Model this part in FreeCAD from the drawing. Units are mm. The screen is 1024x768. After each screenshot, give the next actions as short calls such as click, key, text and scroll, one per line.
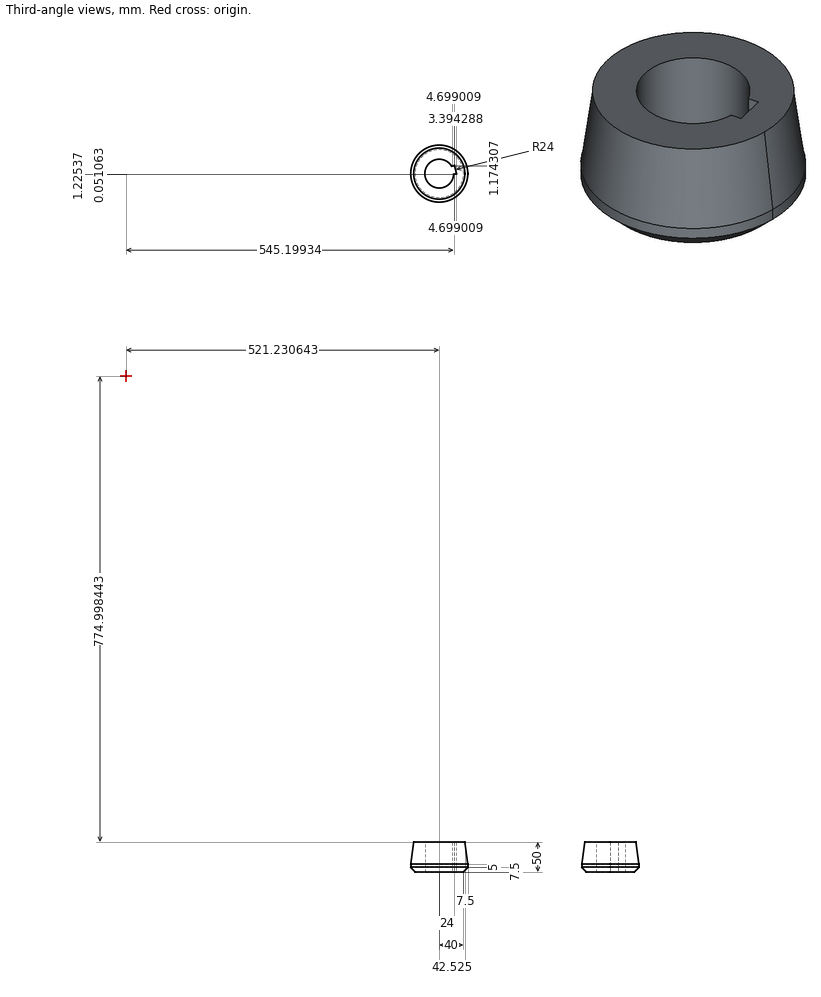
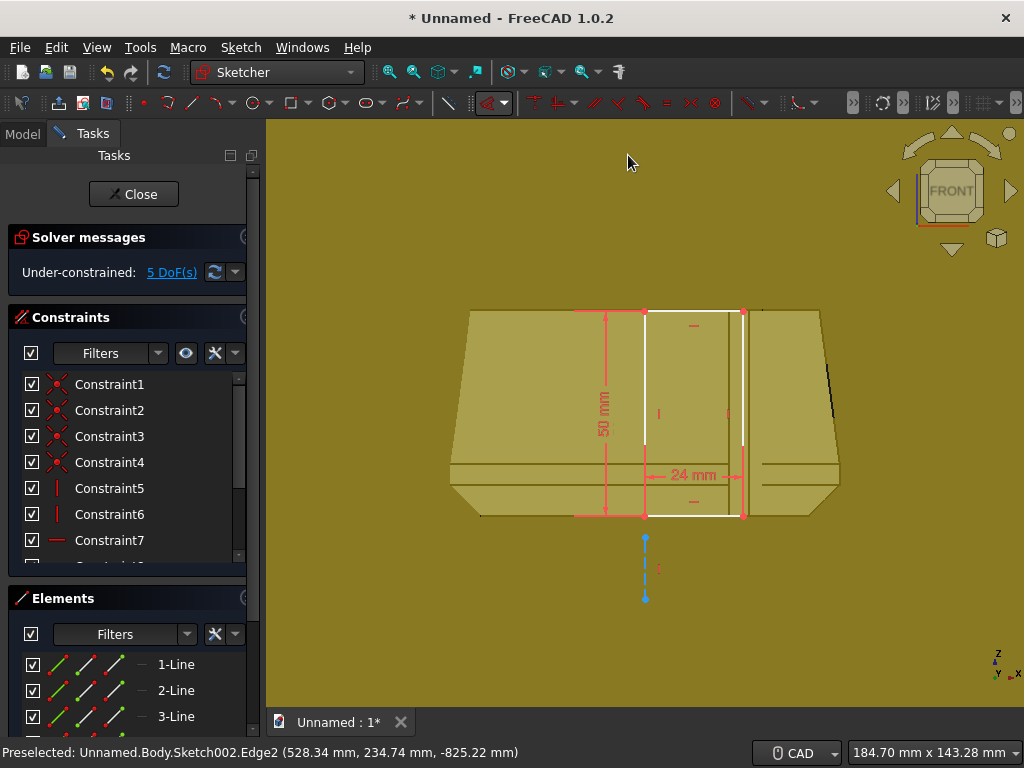
click(645, 311)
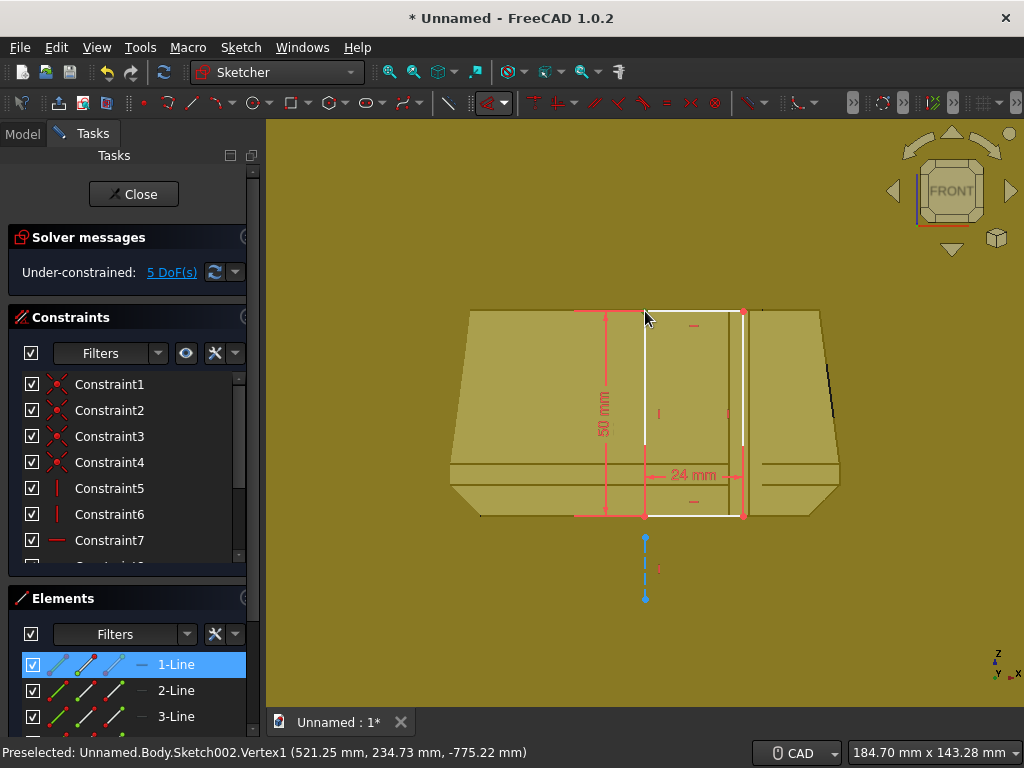
click(506, 104)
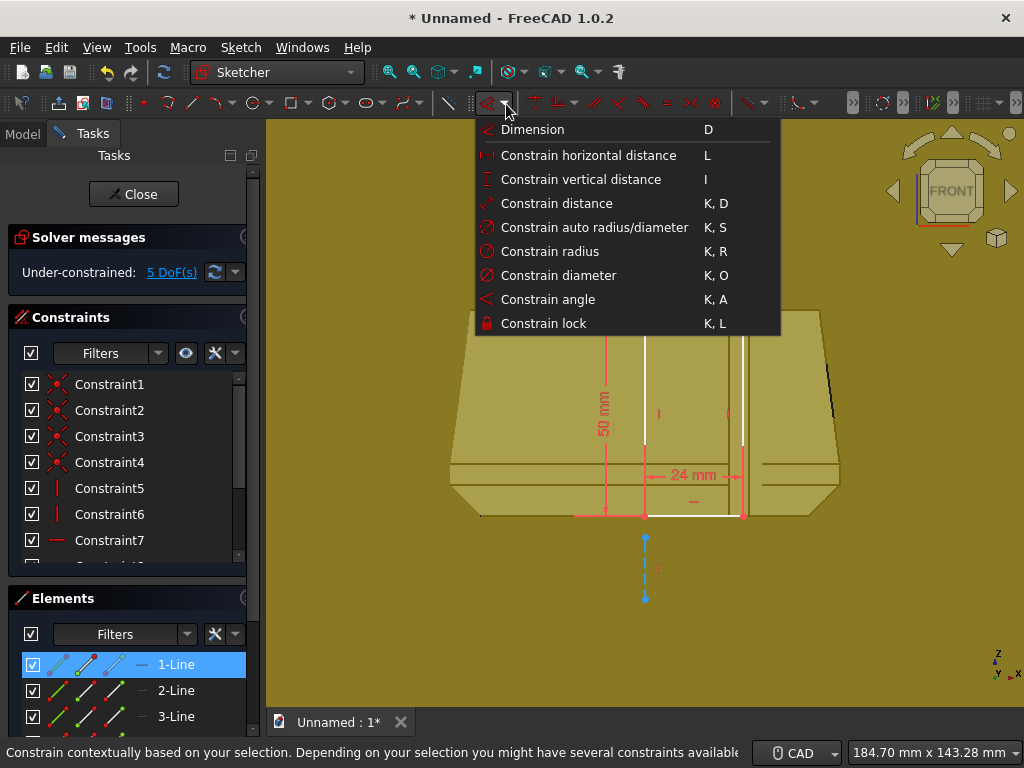
click(628, 155)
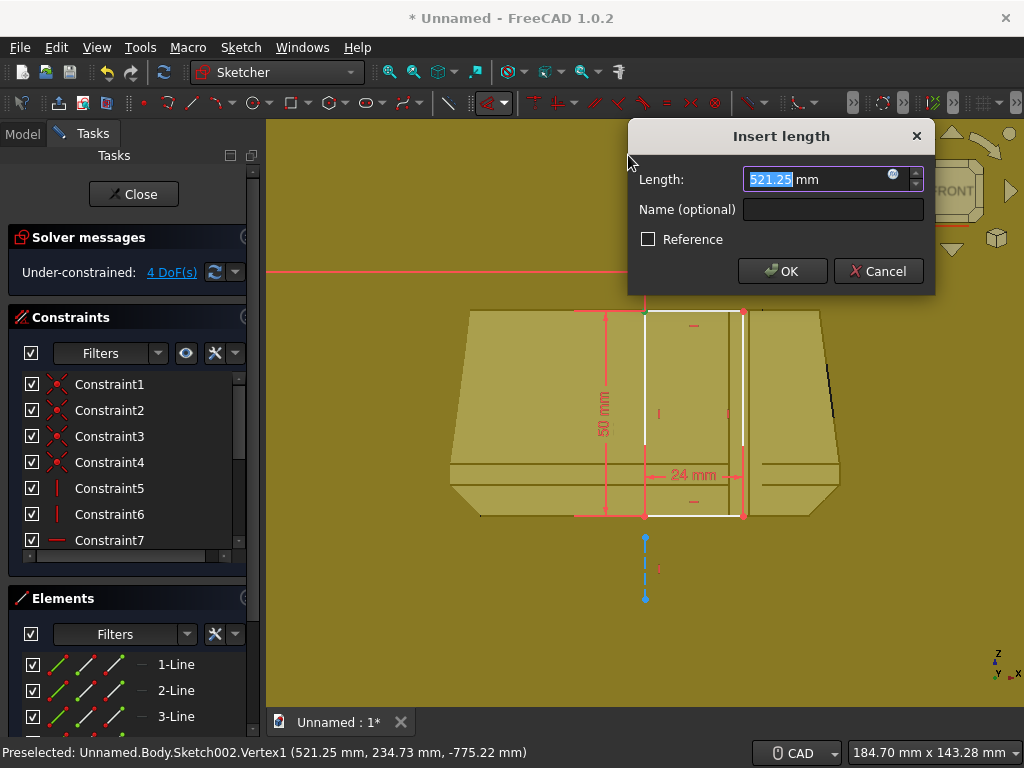
text(521.230643)
key(Return)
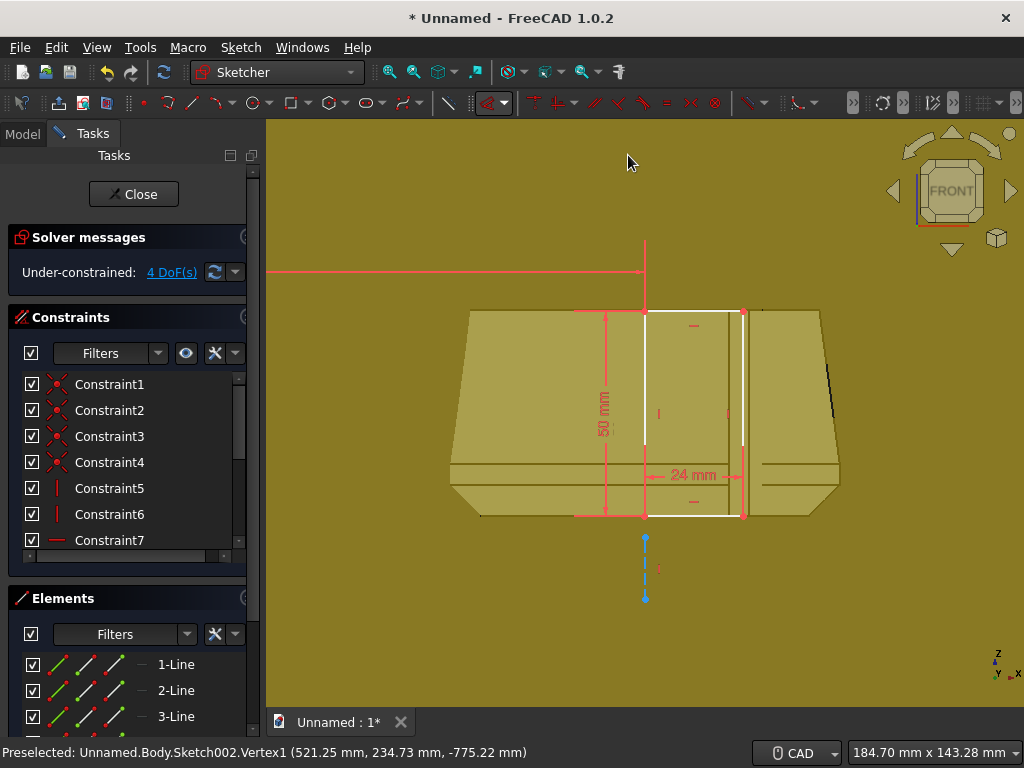
click(645, 311)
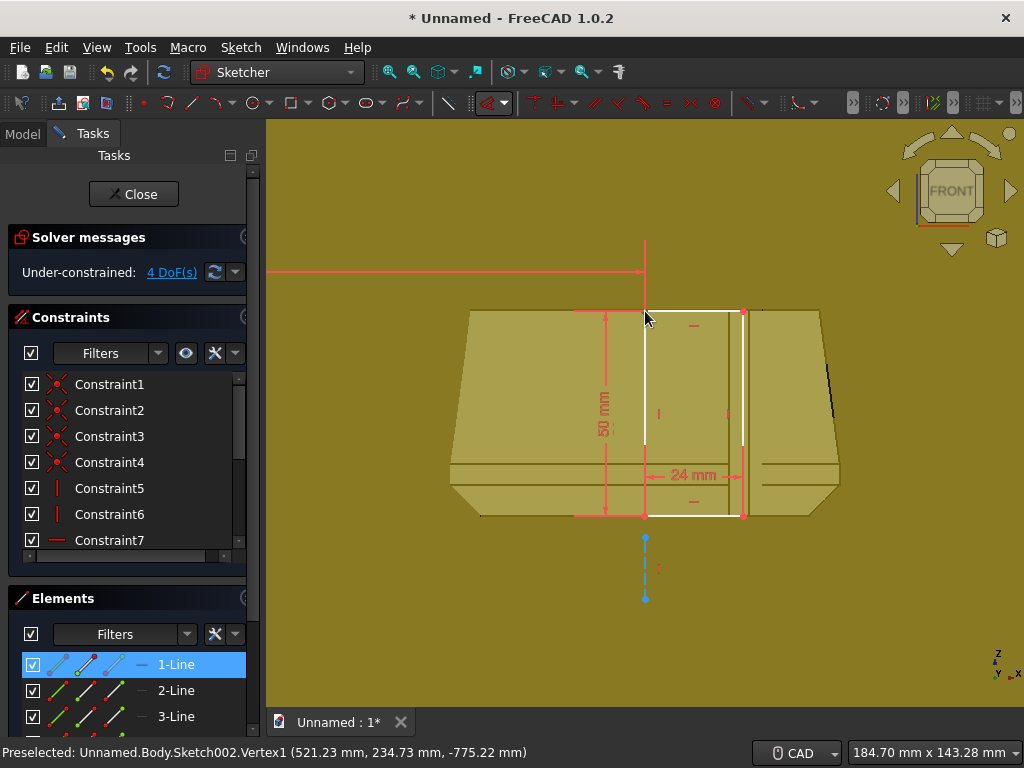
click(506, 104)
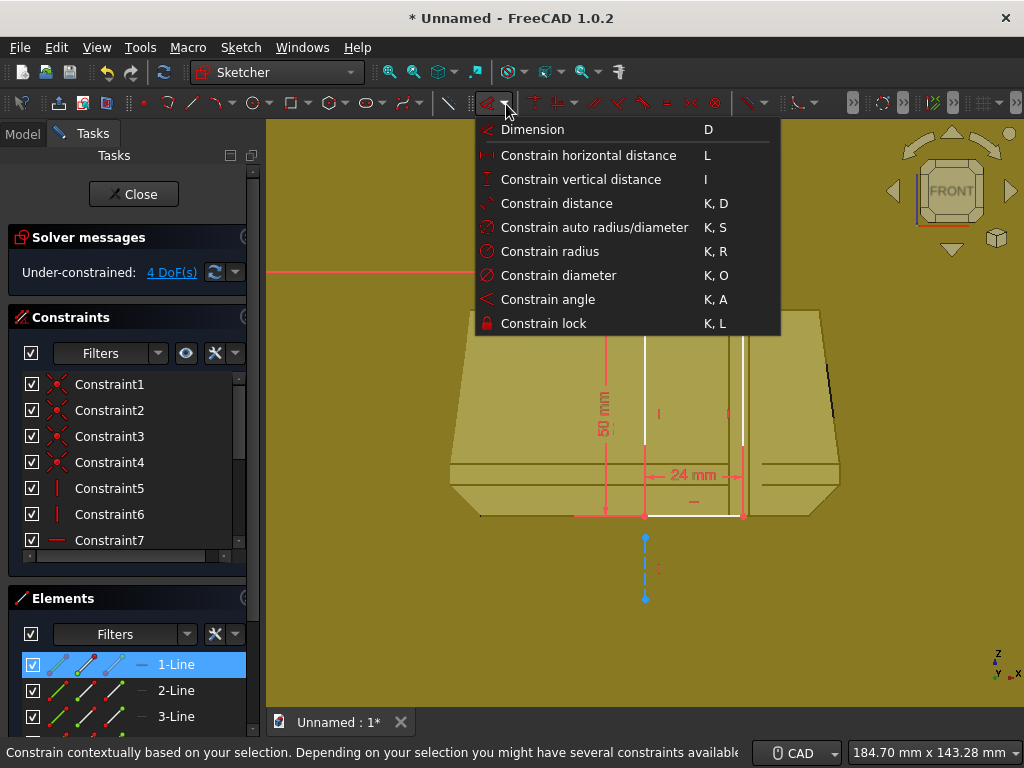
click(628, 179)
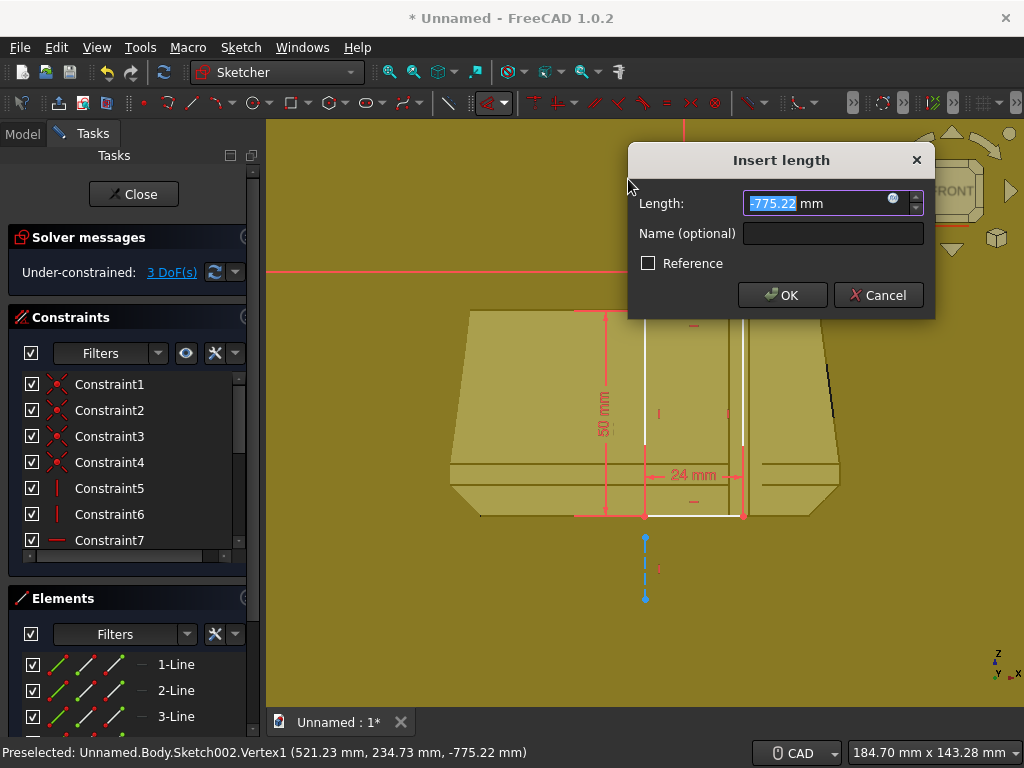
text(-774.998443)
key(Return)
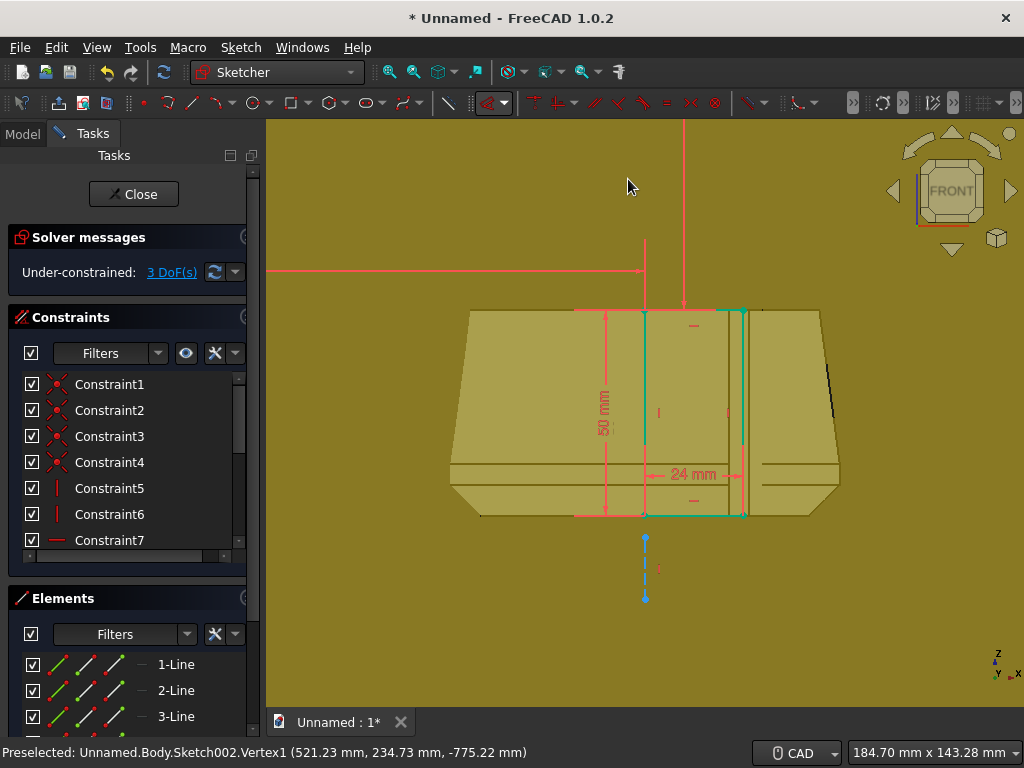
click(645, 537)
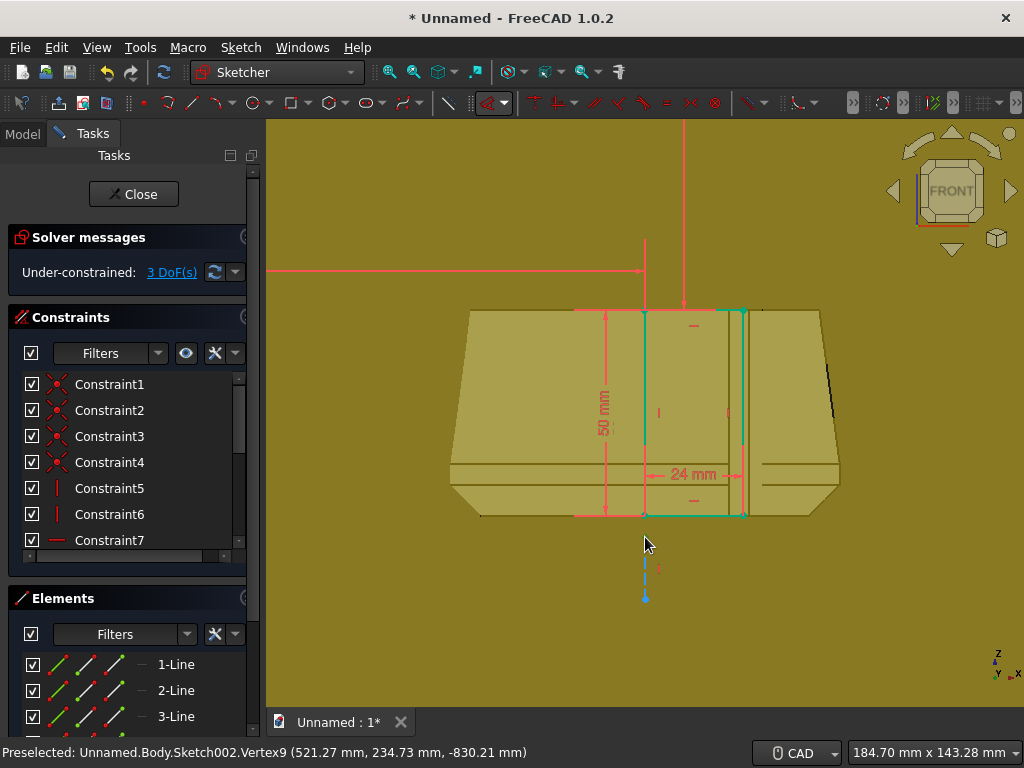
click(506, 104)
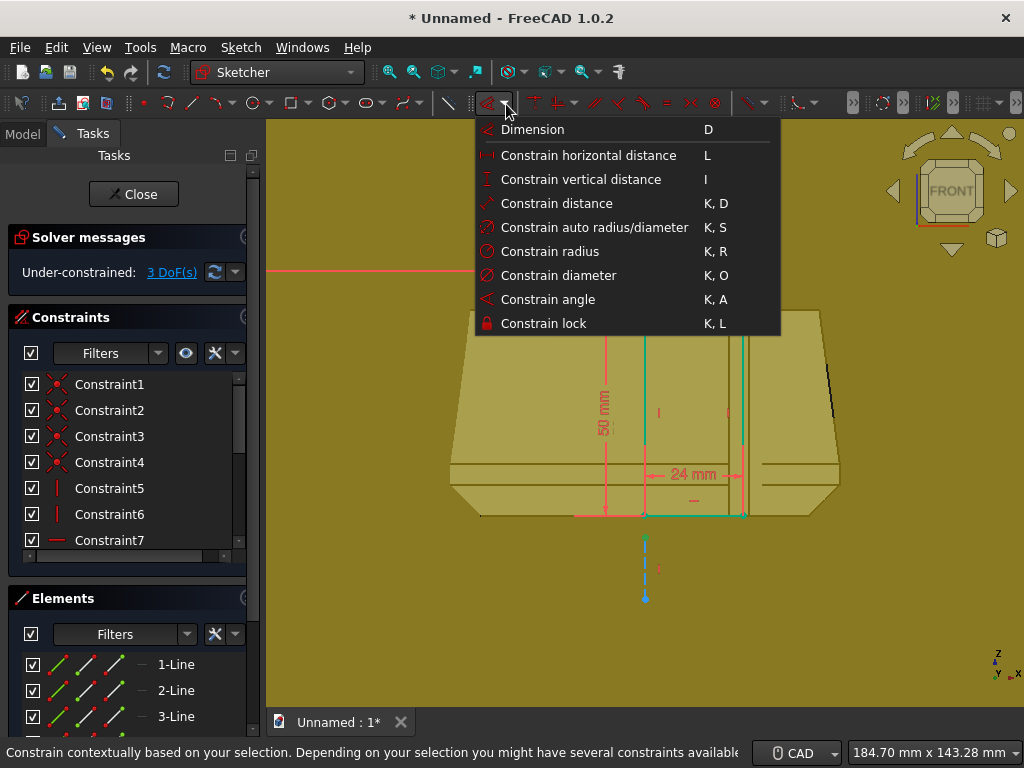
click(628, 155)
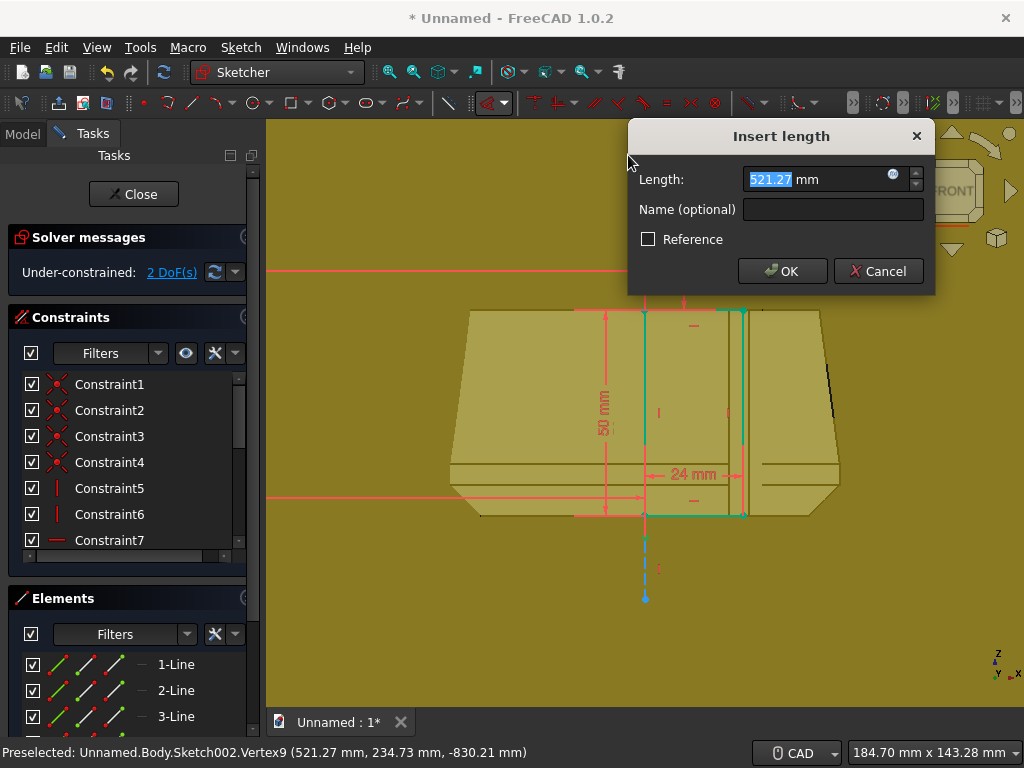
text(521.230643)
key(Return)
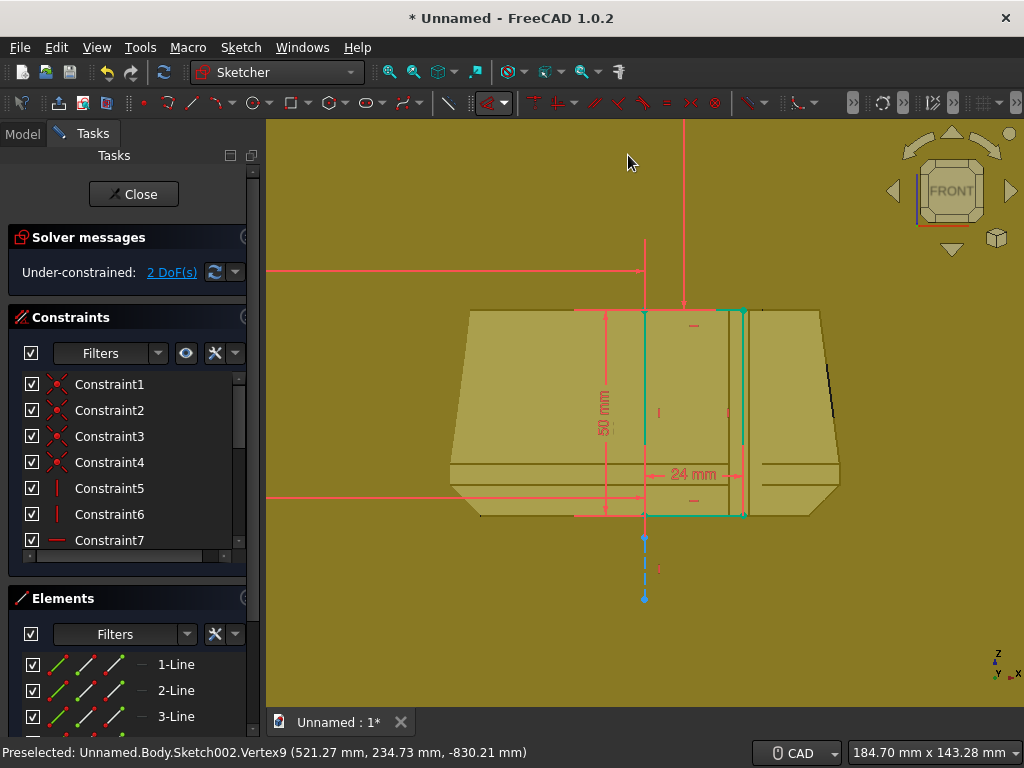
click(134, 194)